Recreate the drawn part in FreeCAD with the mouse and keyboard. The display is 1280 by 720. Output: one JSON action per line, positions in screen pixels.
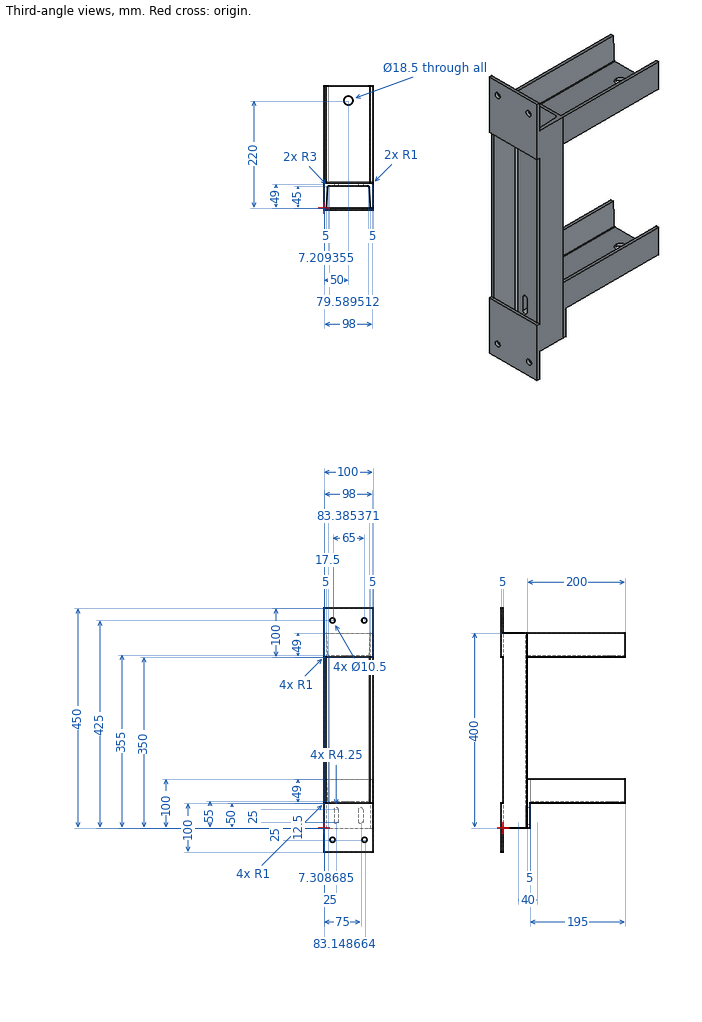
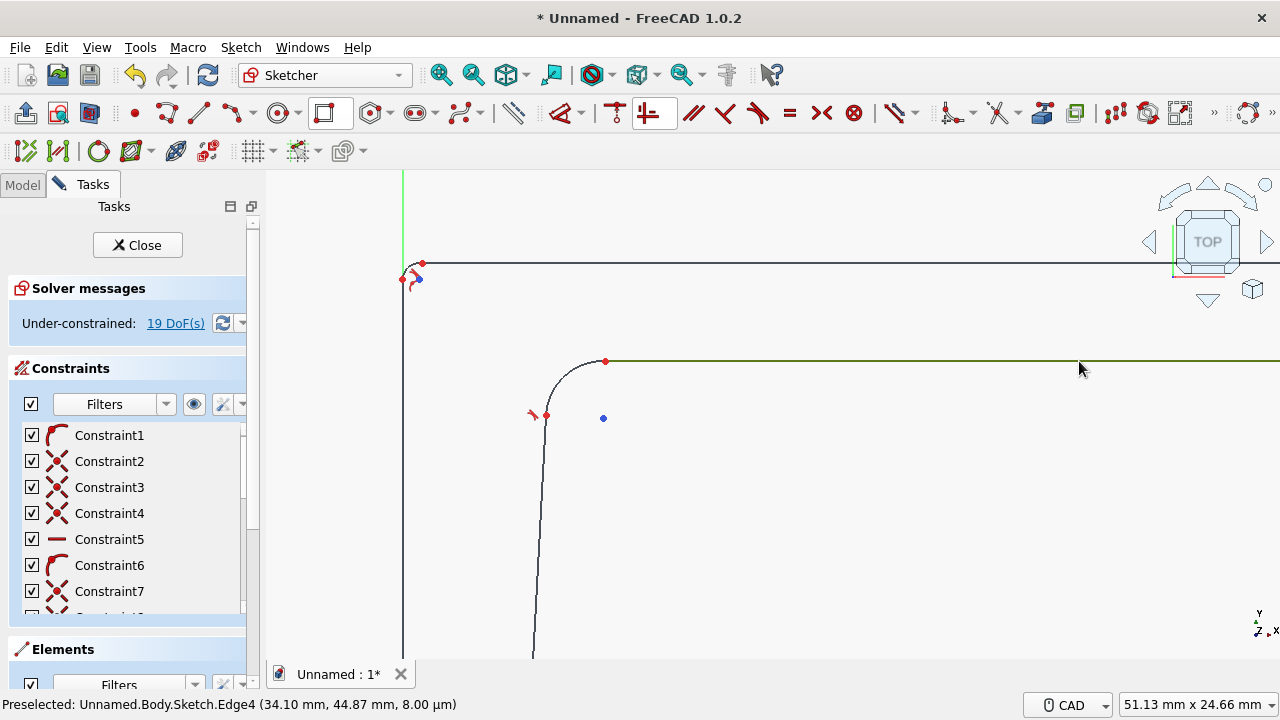
{"action": "left_click", "coordinate": [580, 366]}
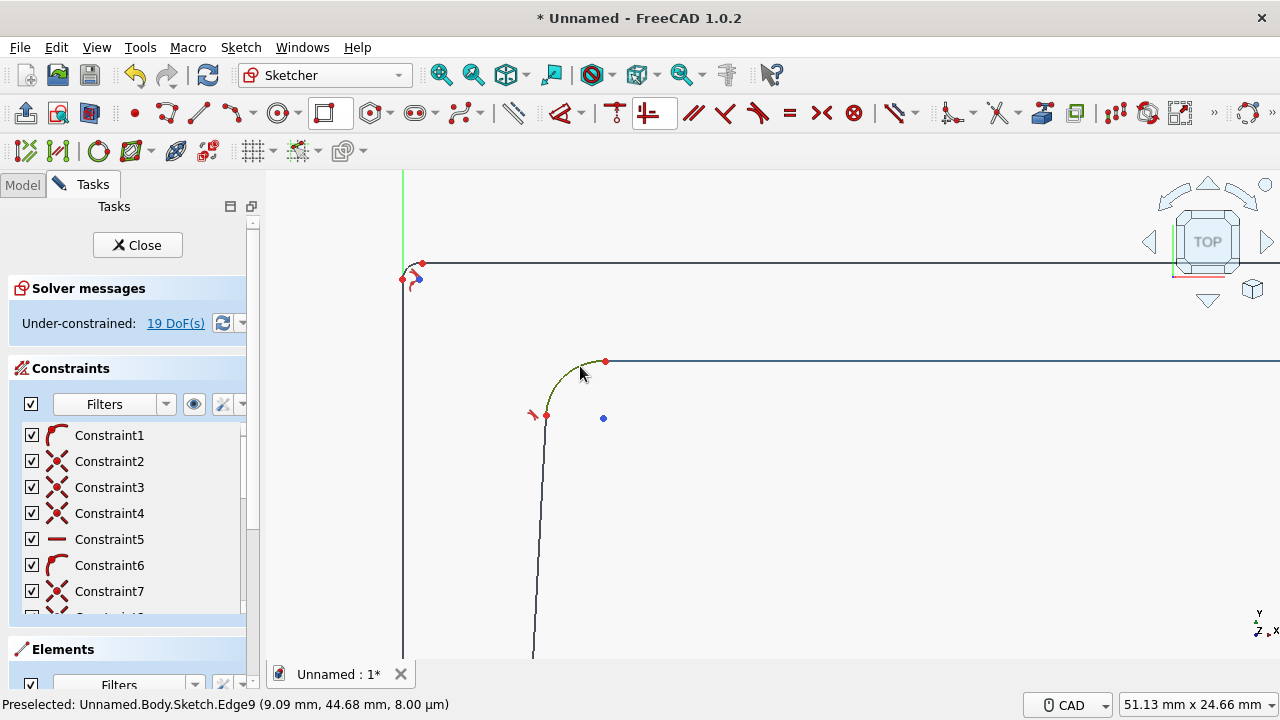
{"action": "left_click", "coordinate": [758, 114]}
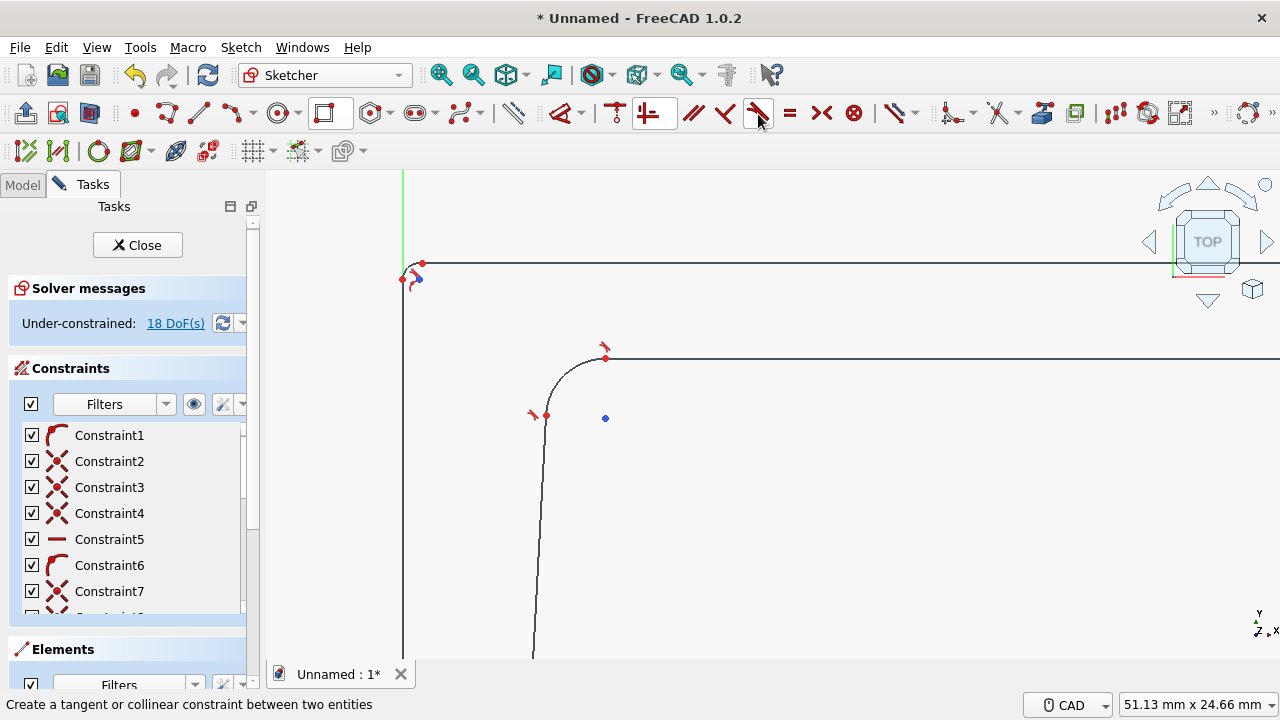
{"action": "left_click", "coordinate": [1079, 359]}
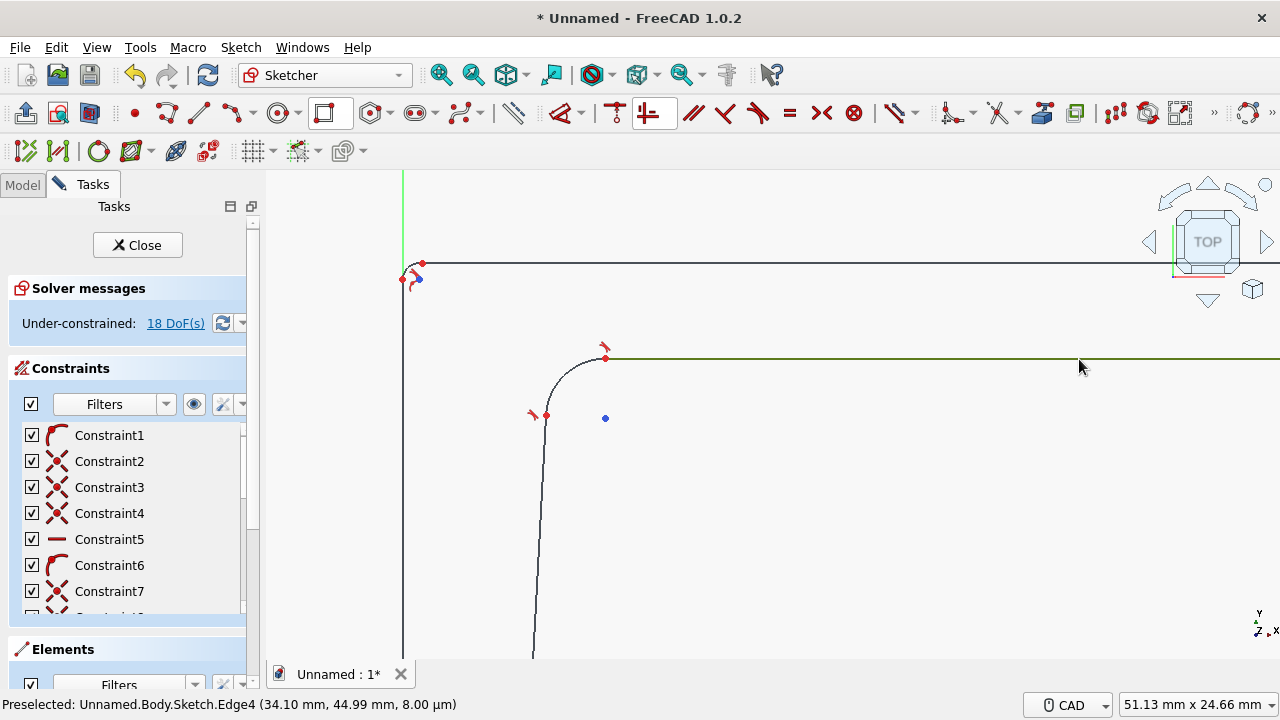
{"action": "scroll", "coordinate": [407, 268], "scroll_direction": "down", "scroll_amount": 6}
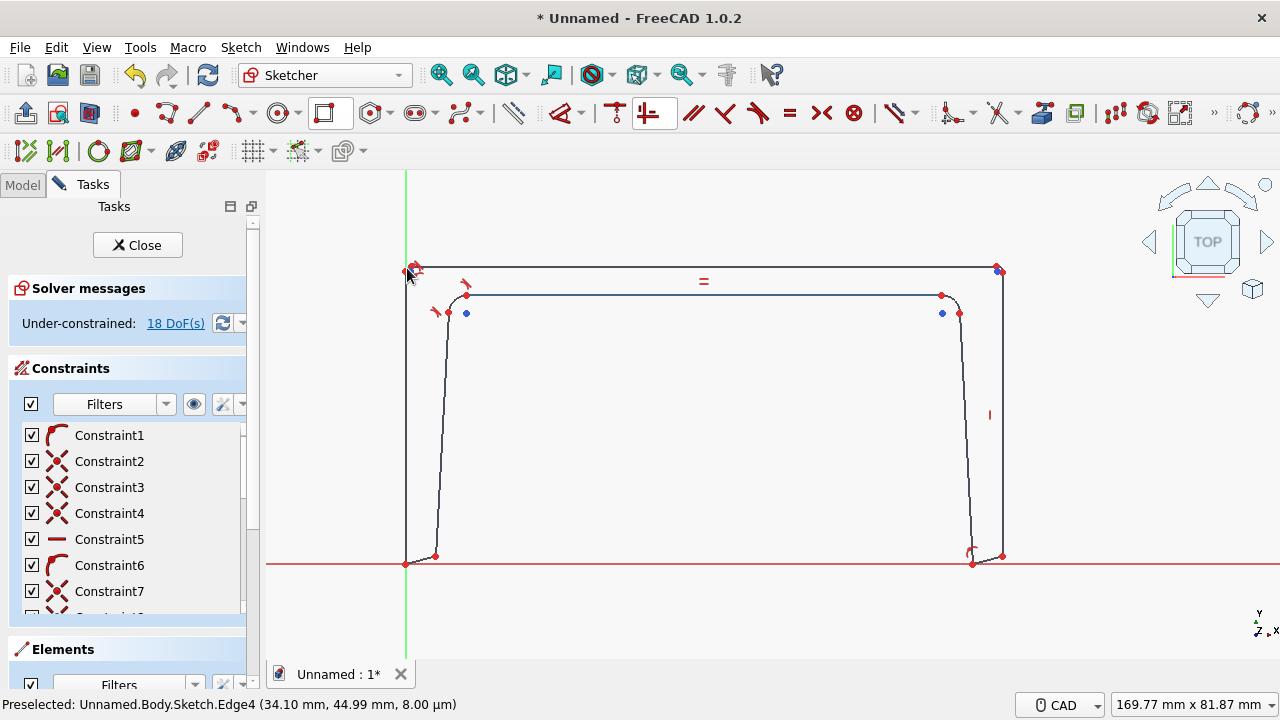
{"action": "scroll", "coordinate": [958, 305], "scroll_direction": "up", "scroll_amount": 3}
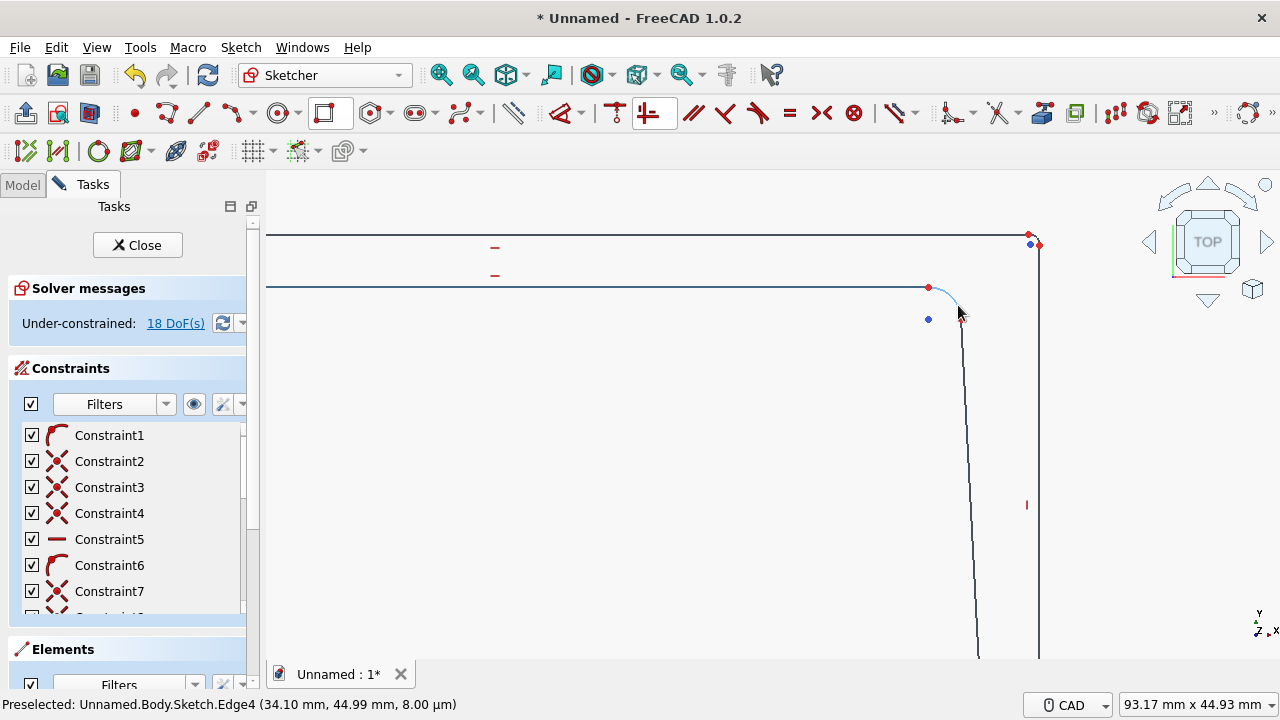
{"action": "left_click", "coordinate": [957, 305]}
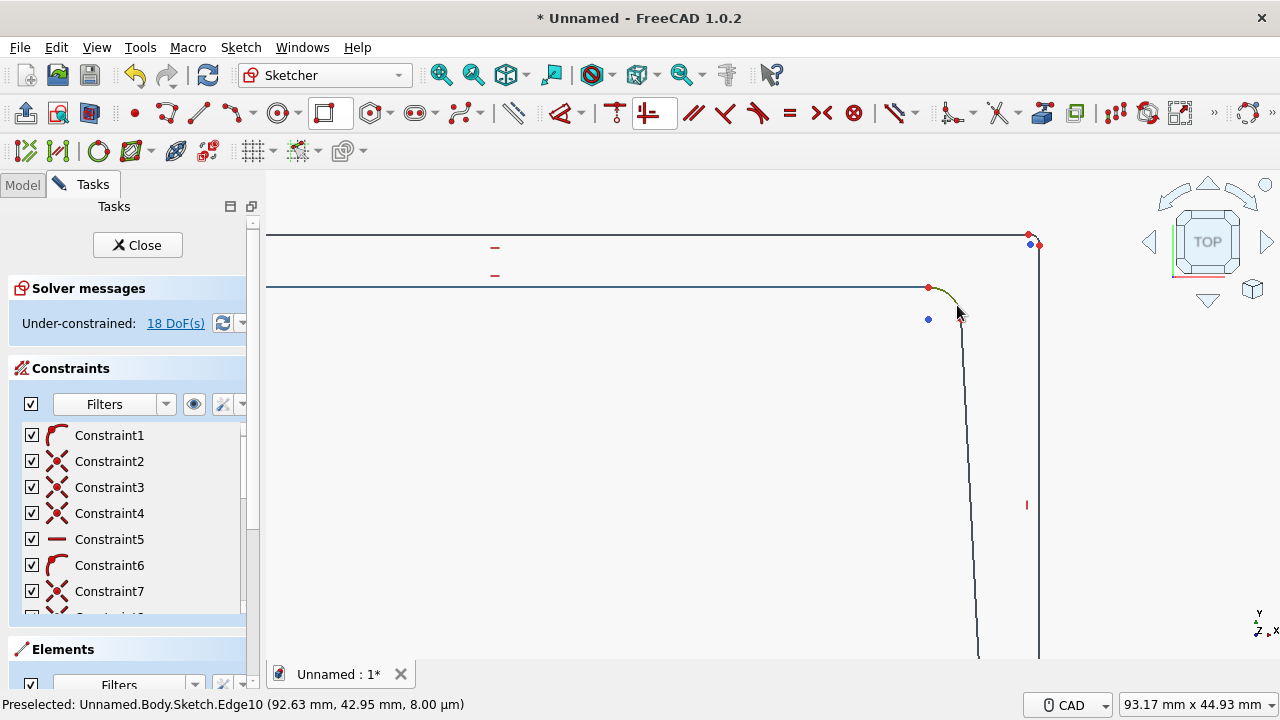
{"action": "left_click", "coordinate": [758, 114]}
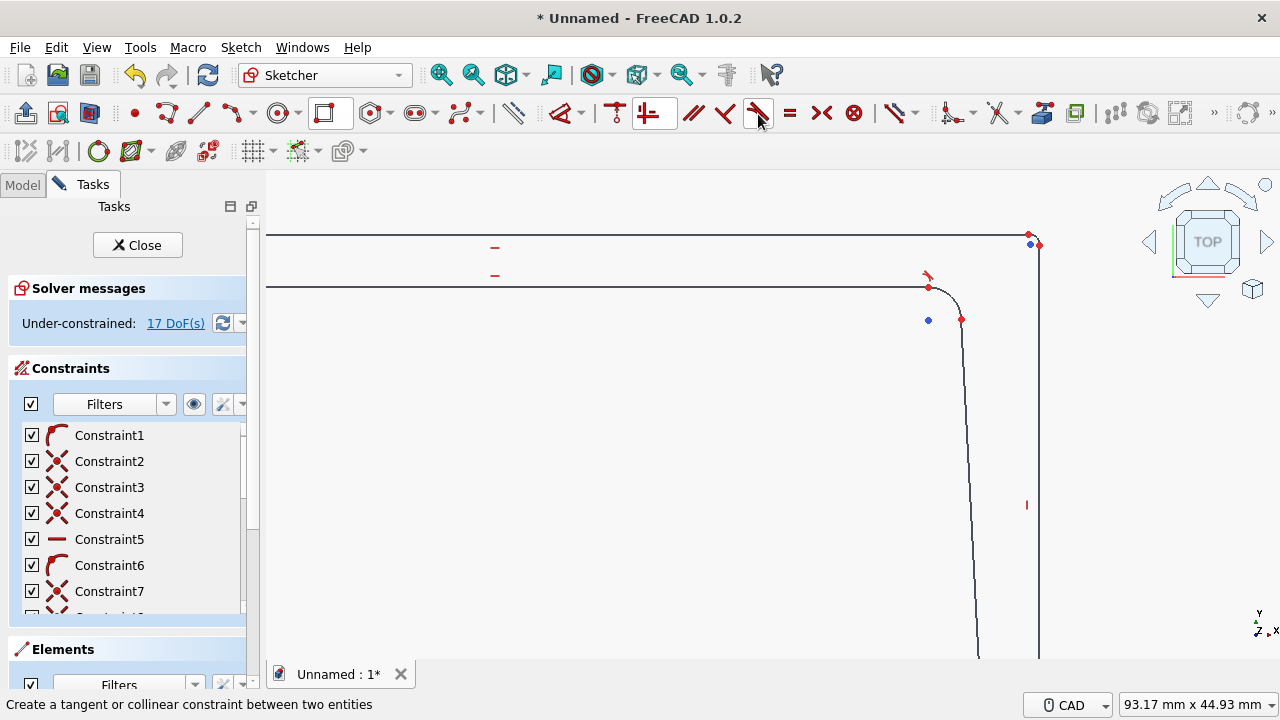
{"action": "left_click", "coordinate": [968, 457]}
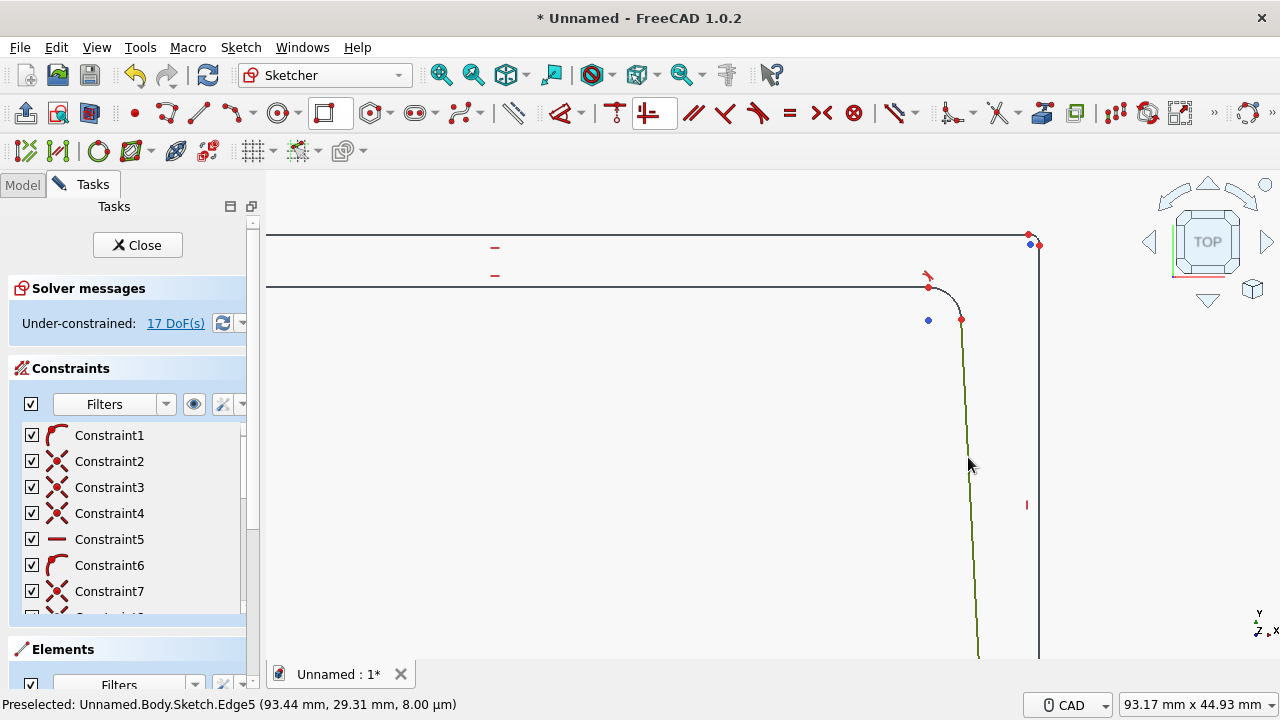
{"action": "left_click", "coordinate": [957, 305]}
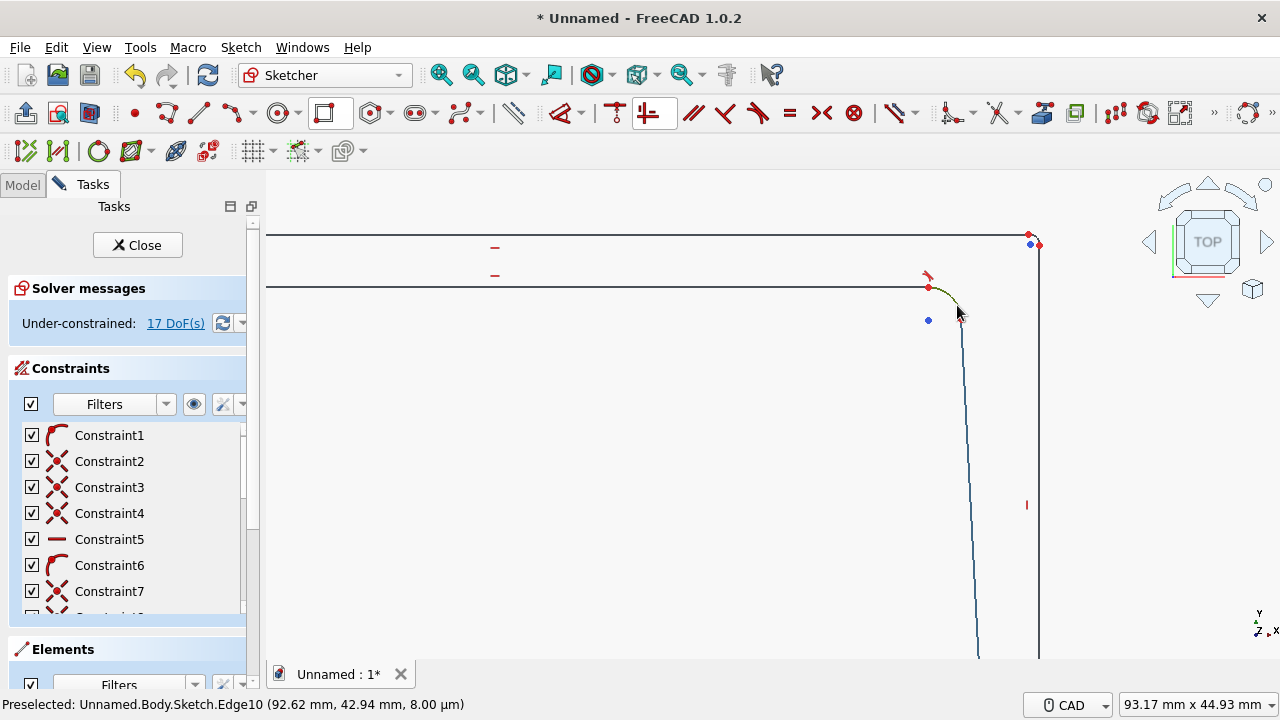
{"action": "left_click", "coordinate": [758, 114]}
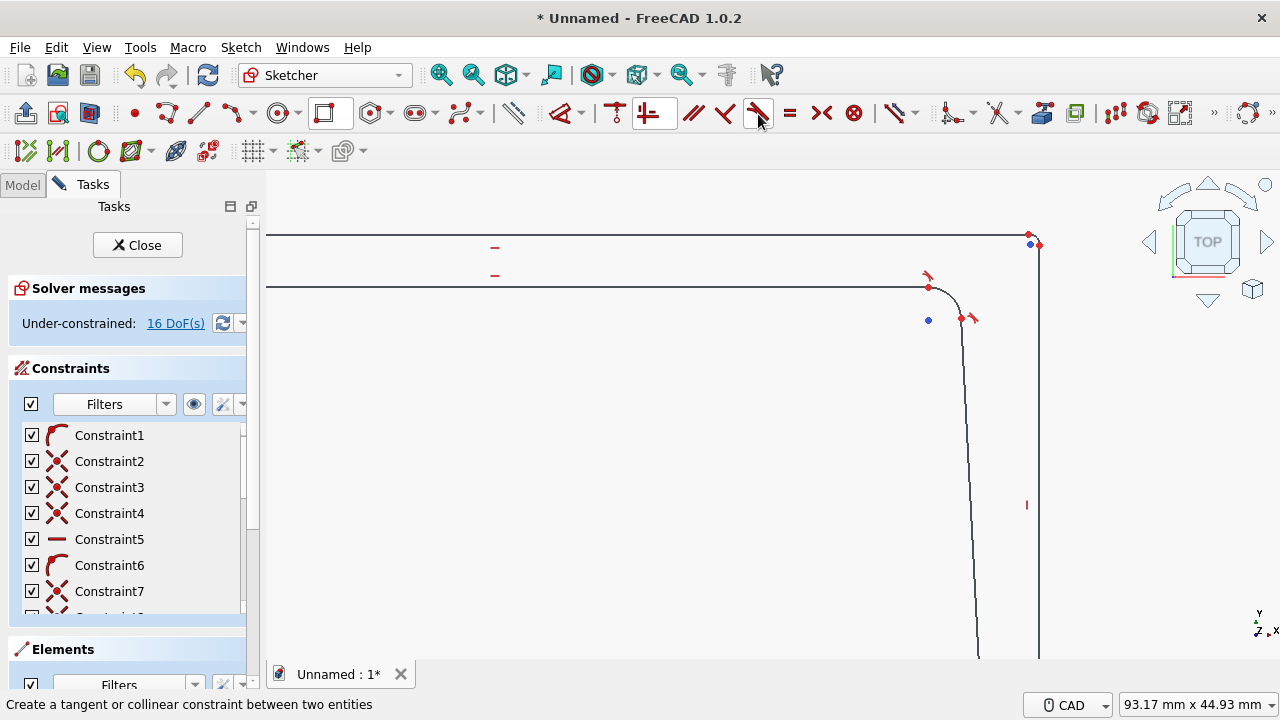
{"action": "left_click", "coordinate": [1039, 607]}